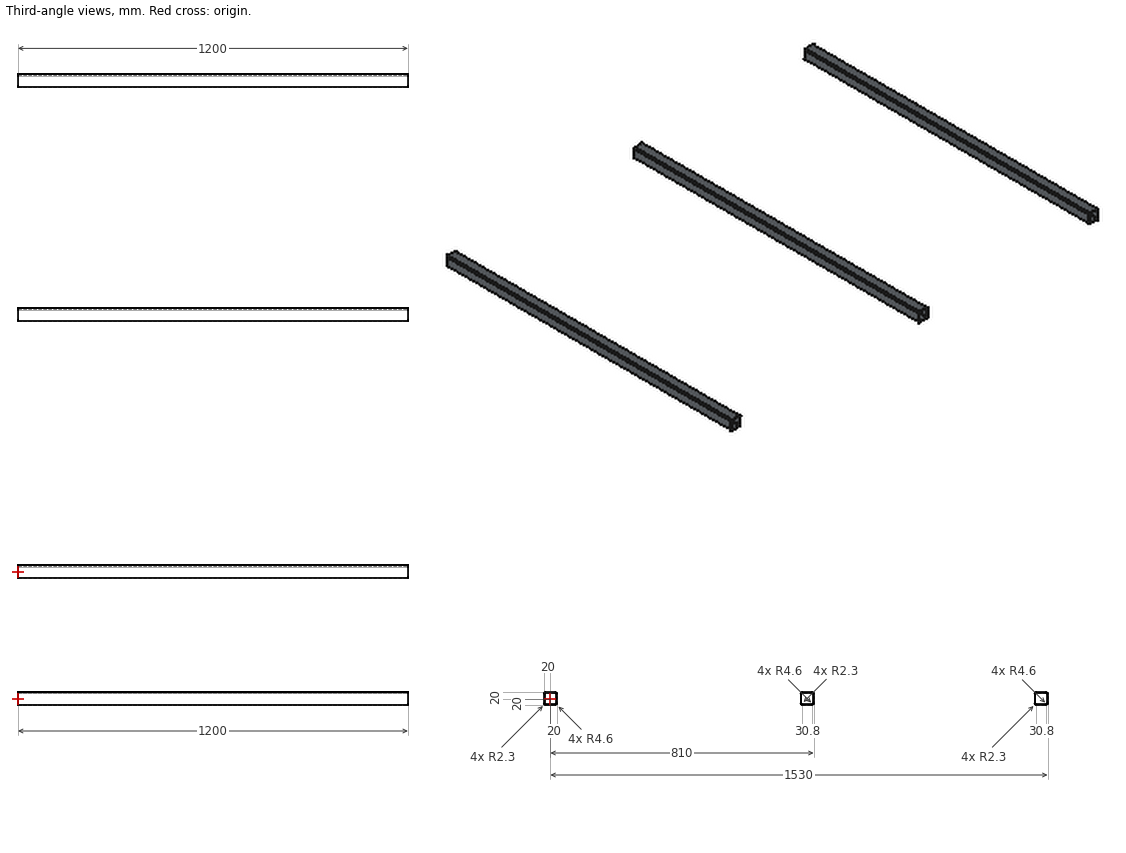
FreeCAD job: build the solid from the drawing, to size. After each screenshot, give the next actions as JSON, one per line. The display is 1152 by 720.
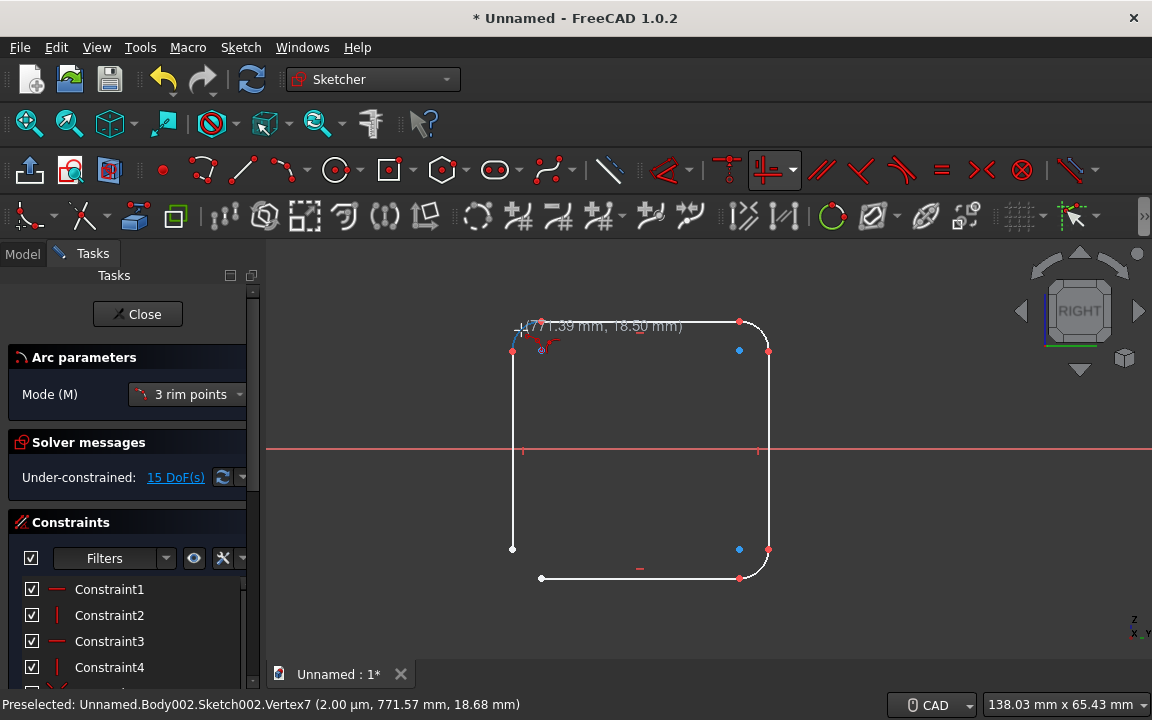
{"action": "left_click", "coordinate": [513, 550]}
{"action": "left_click", "coordinate": [542, 579]}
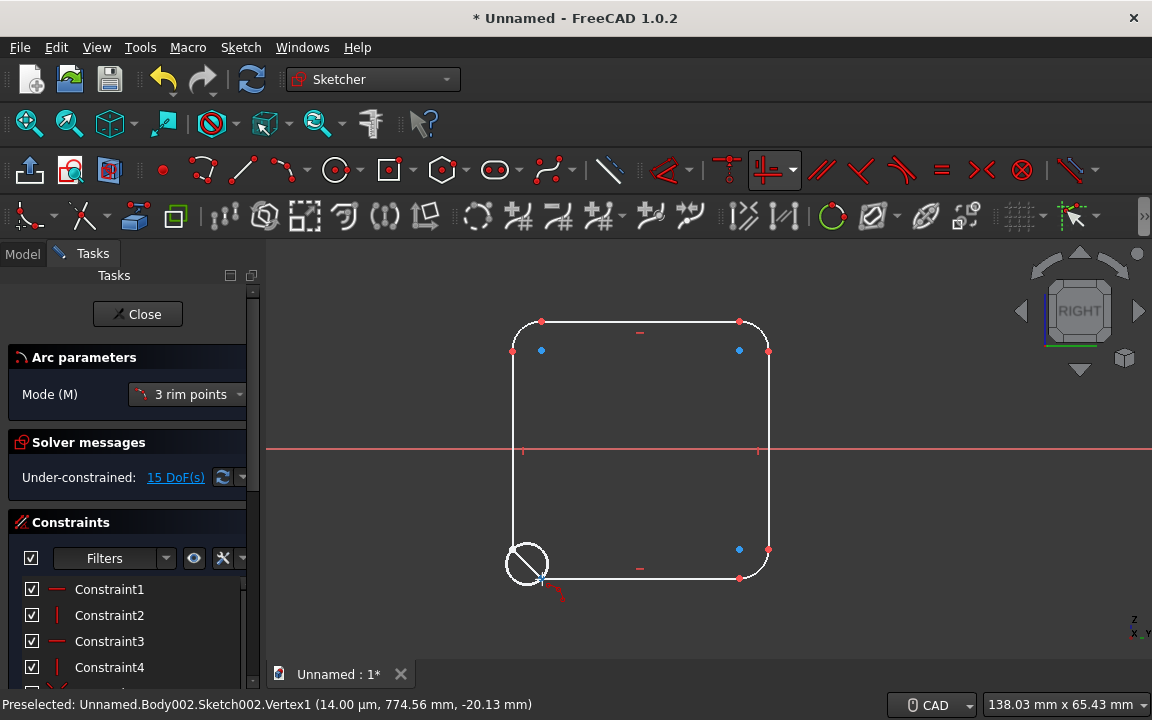
{"action": "scroll", "coordinate": [521, 569], "scroll_direction": "up", "scroll_amount": 4}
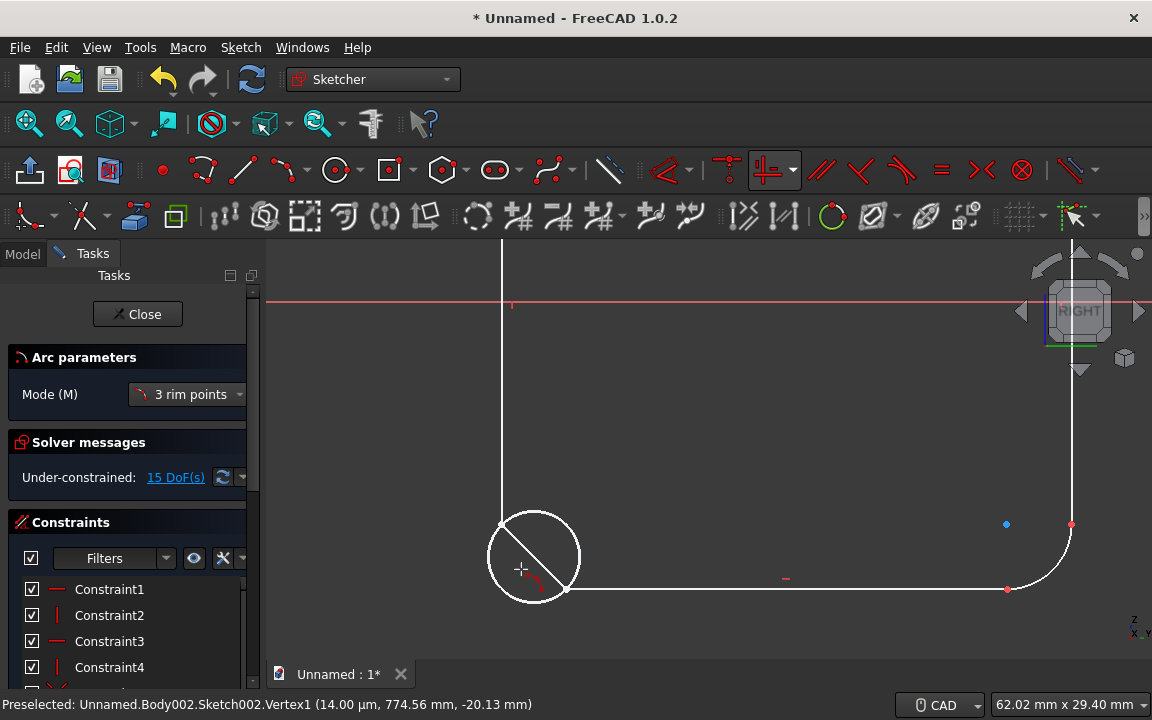
{"action": "left_click", "coordinate": [520, 568]}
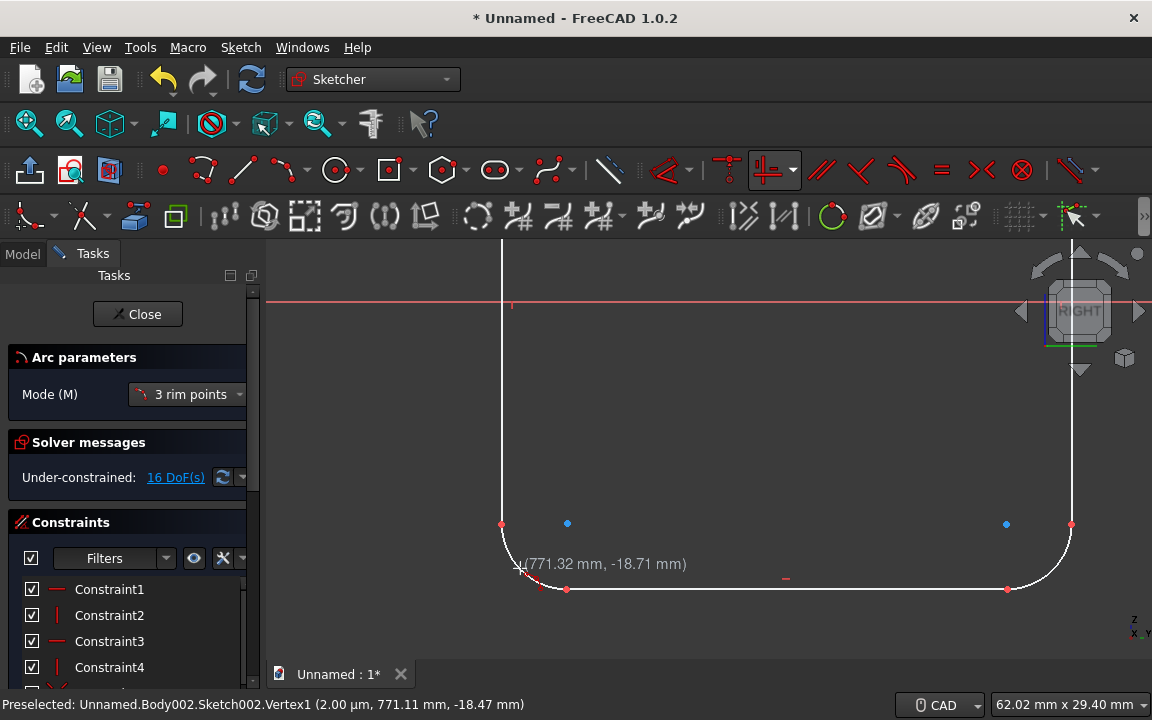
{"action": "key", "text": "g l"}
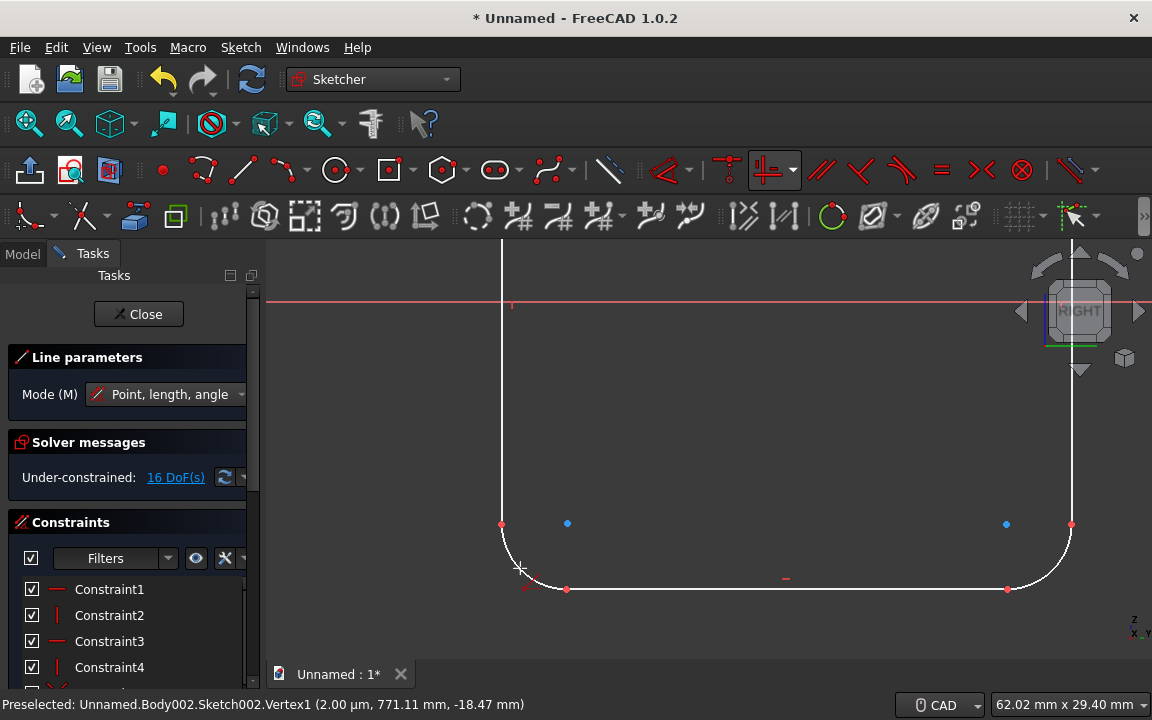
{"action": "scroll", "coordinate": [521, 569], "scroll_direction": "down", "scroll_amount": 4}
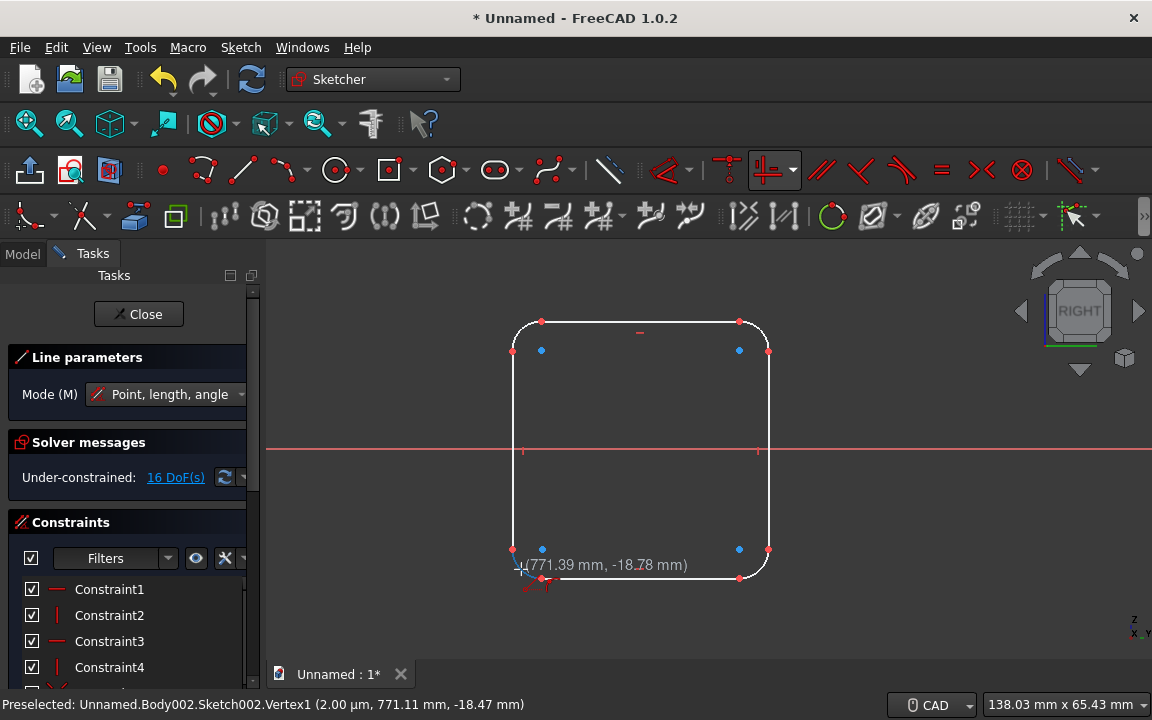
{"action": "left_click", "coordinate": [739, 563]}
{"action": "left_click", "coordinate": [542, 563]}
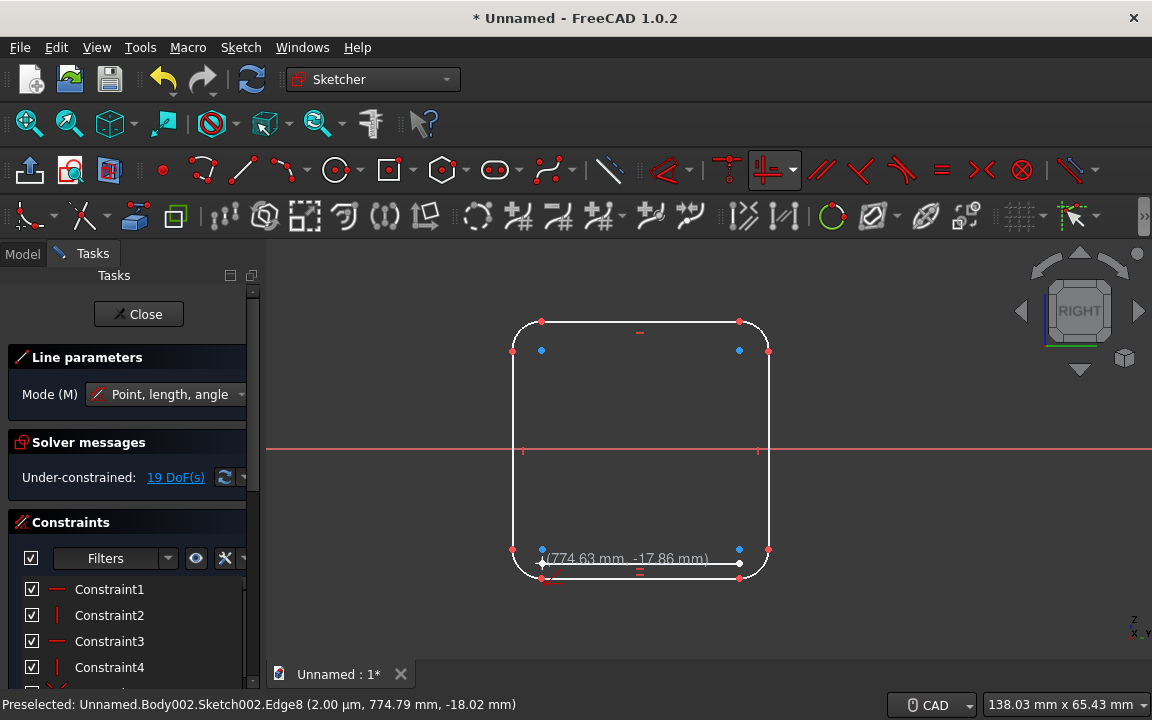
{"action": "left_click", "coordinate": [527, 548]}
{"action": "left_click", "coordinate": [527, 350]}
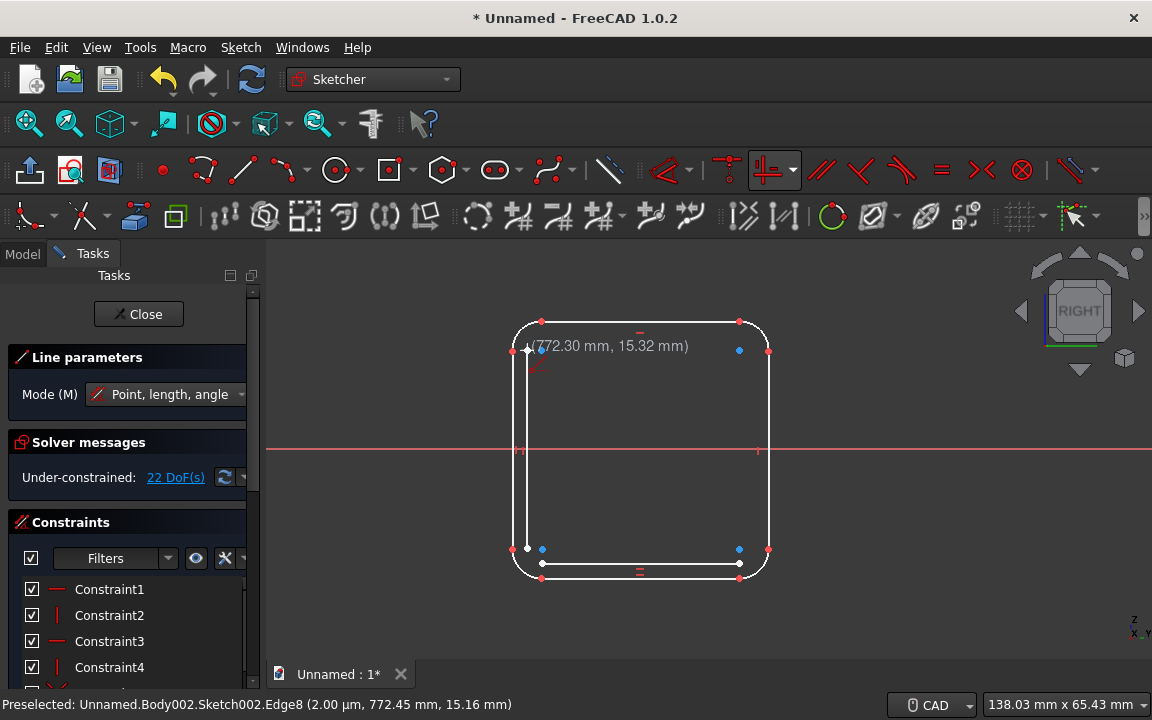
{"action": "left_click", "coordinate": [542, 336]}
{"action": "left_click", "coordinate": [739, 336]}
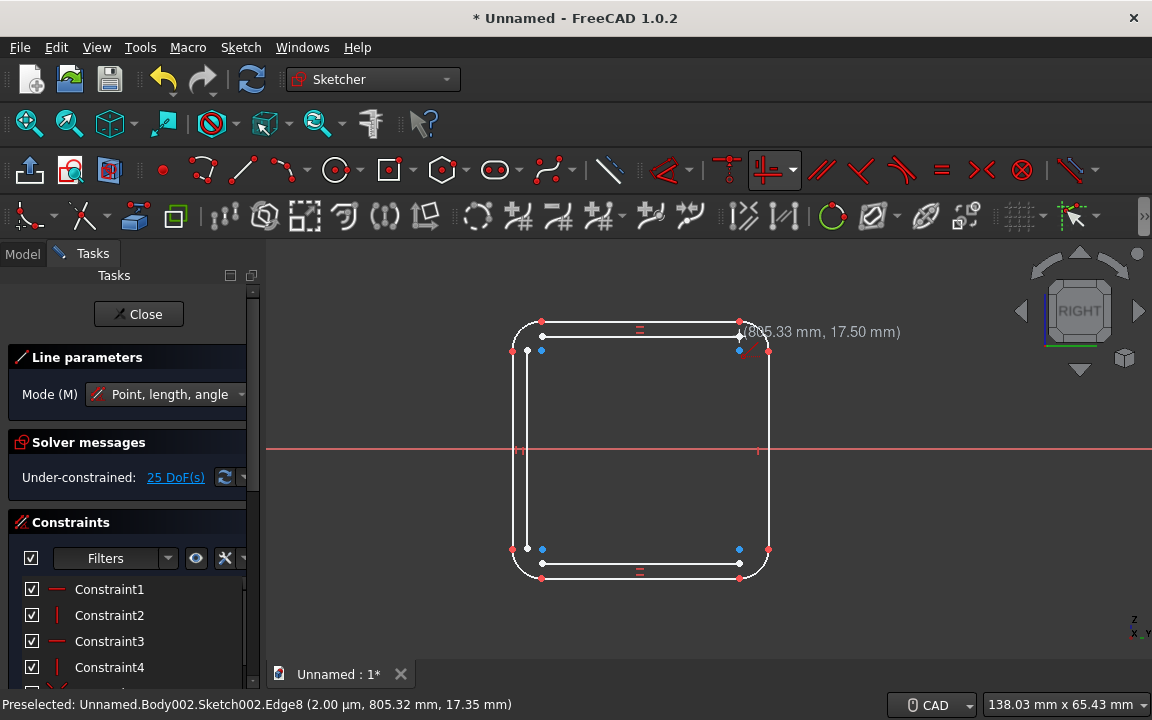
{"action": "left_click", "coordinate": [754, 350]}
{"action": "left_click", "coordinate": [754, 548]}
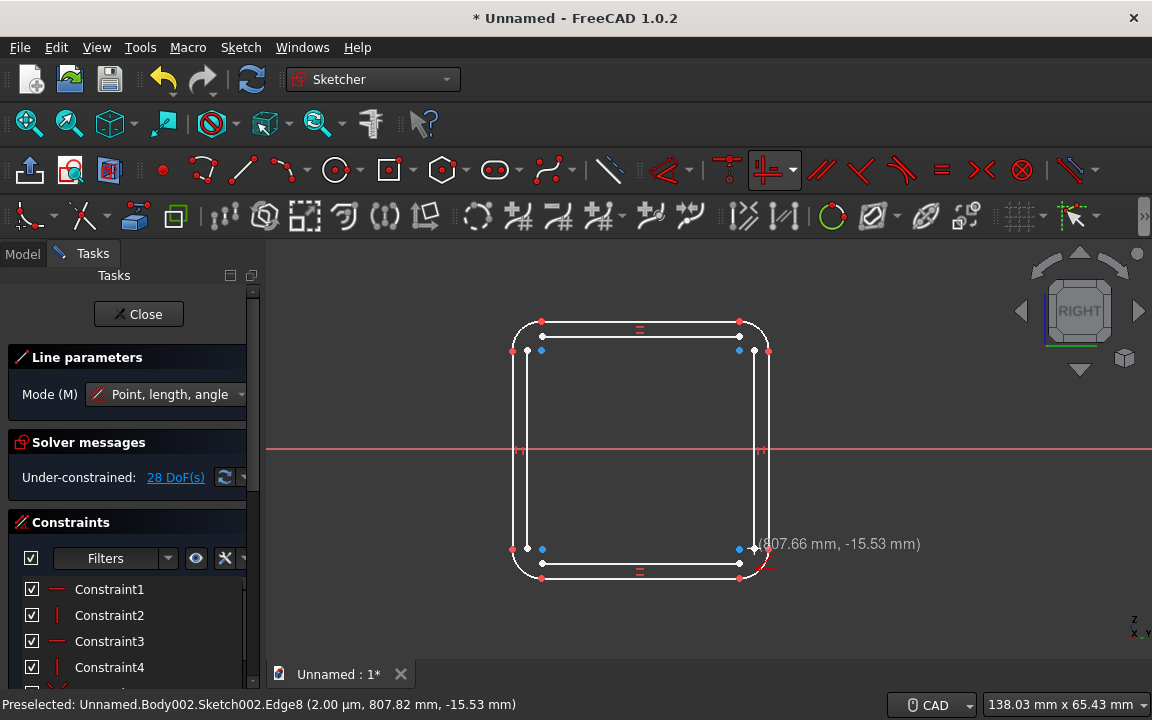
{"action": "key", "text": "g 3 a"}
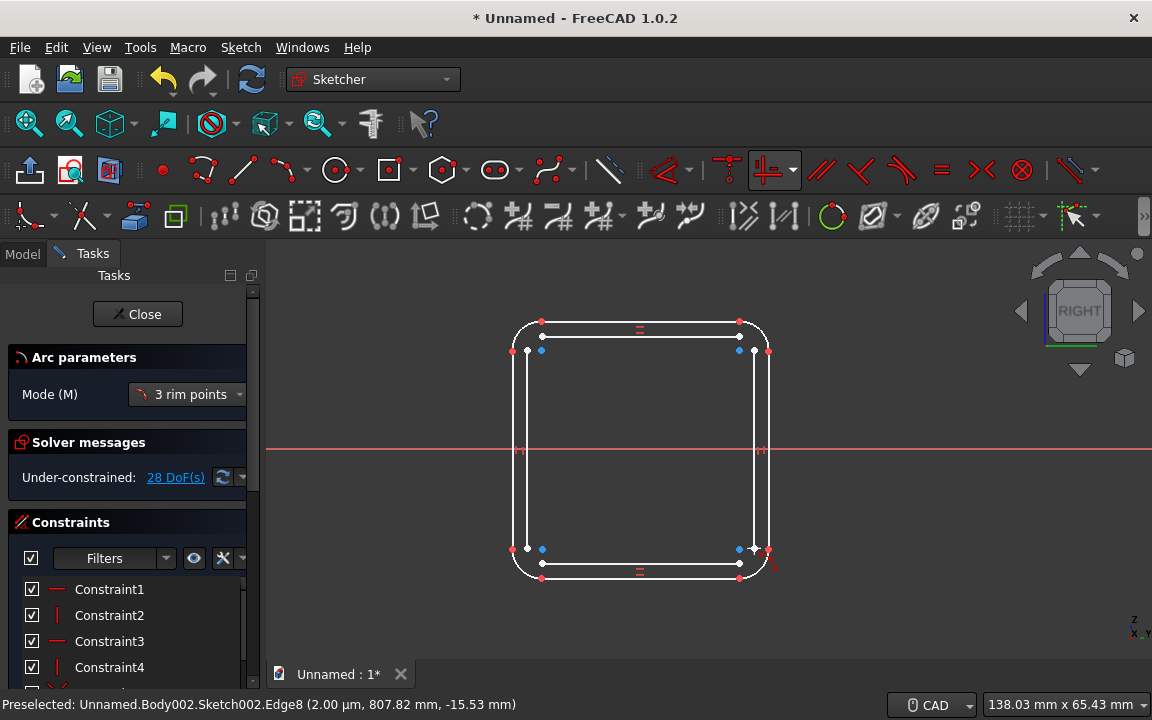
{"action": "left_click", "coordinate": [542, 564]}
{"action": "left_click", "coordinate": [527, 549]}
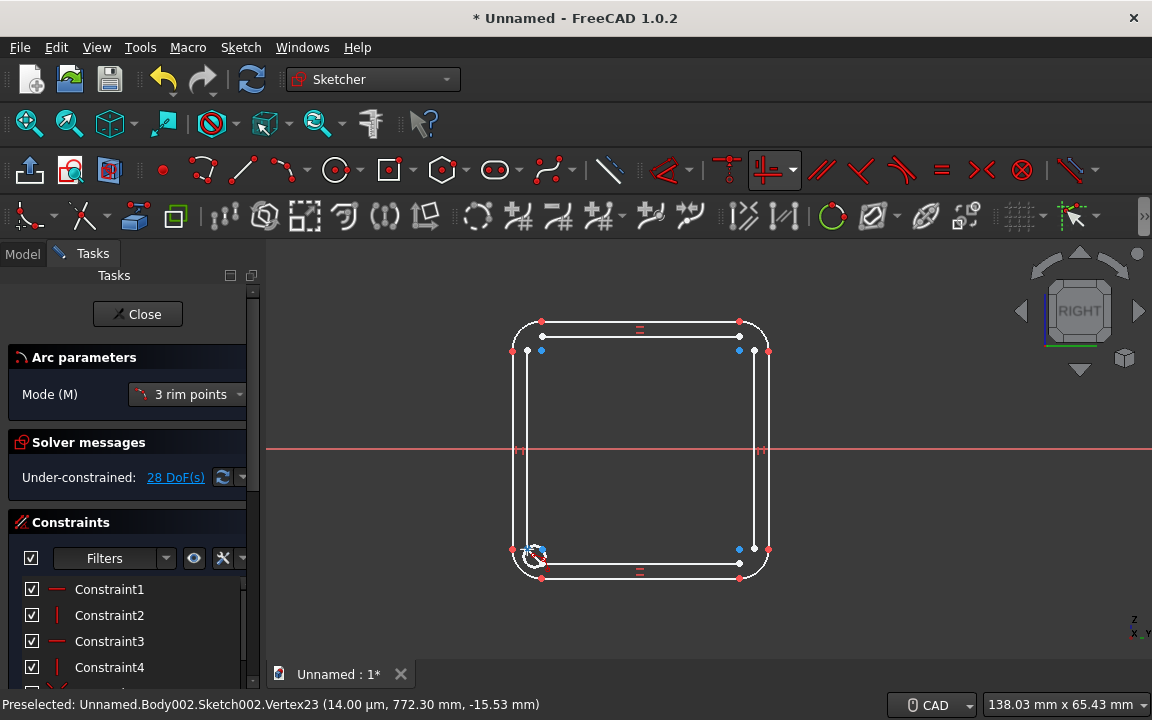
{"action": "scroll", "coordinate": [531, 559], "scroll_direction": "up", "scroll_amount": 7}